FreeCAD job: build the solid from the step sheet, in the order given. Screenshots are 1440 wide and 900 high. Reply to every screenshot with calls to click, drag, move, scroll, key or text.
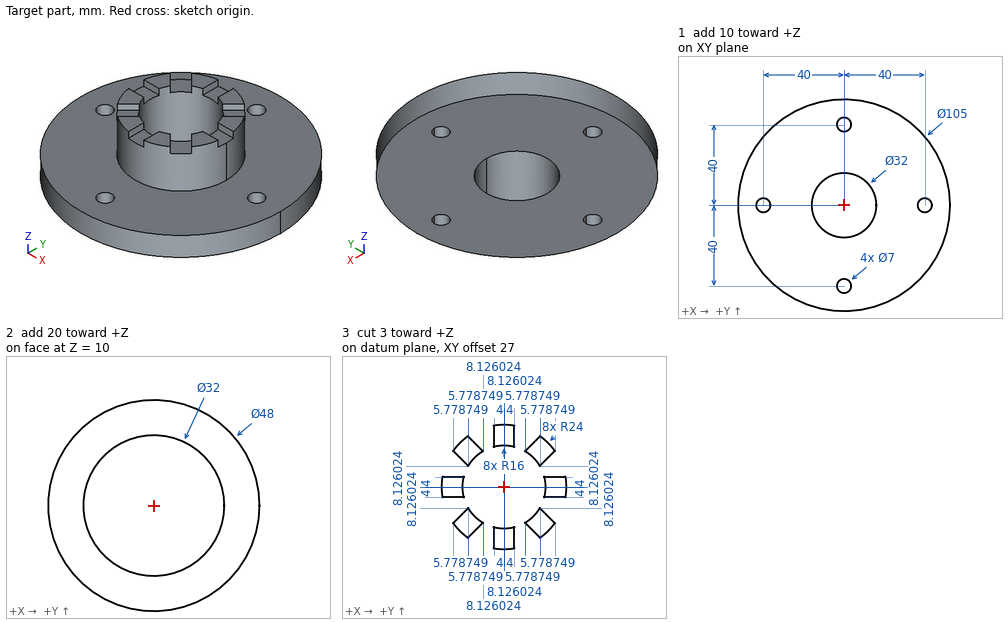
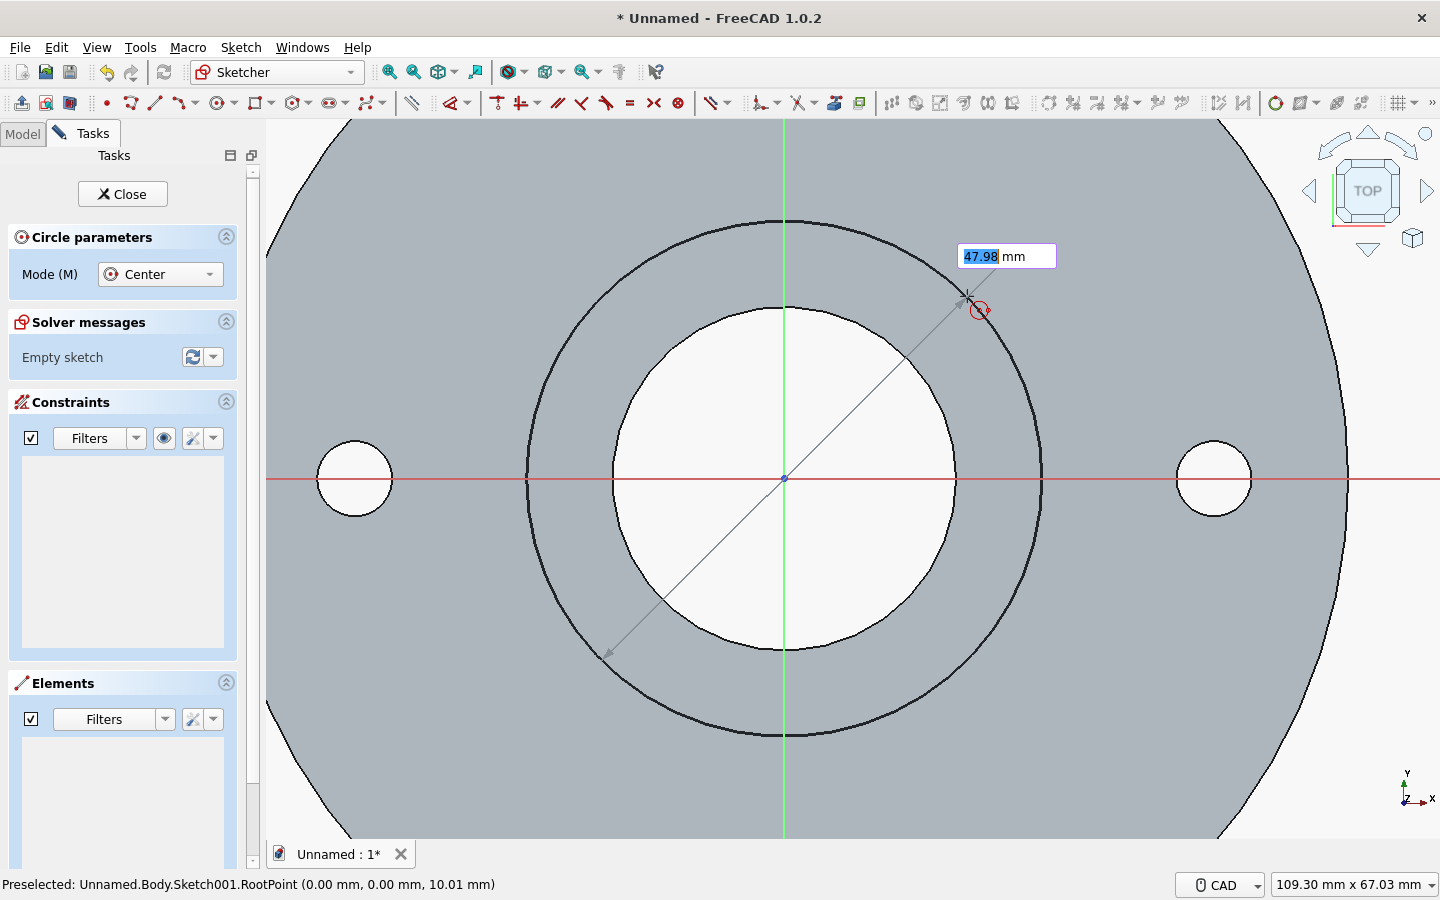
text(48)
key(Return)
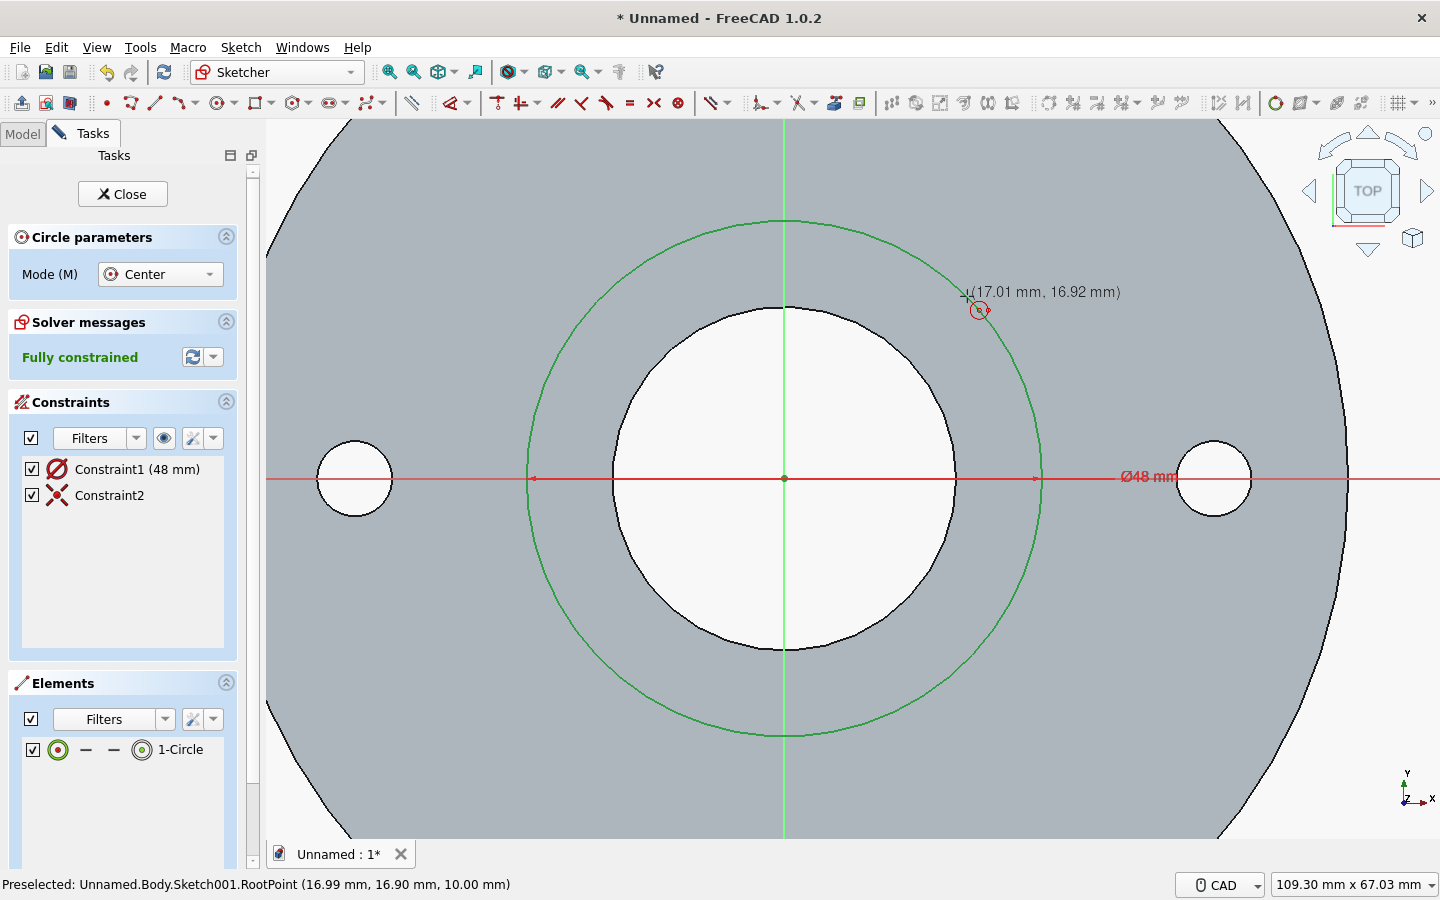
click(784, 479)
move(906, 357)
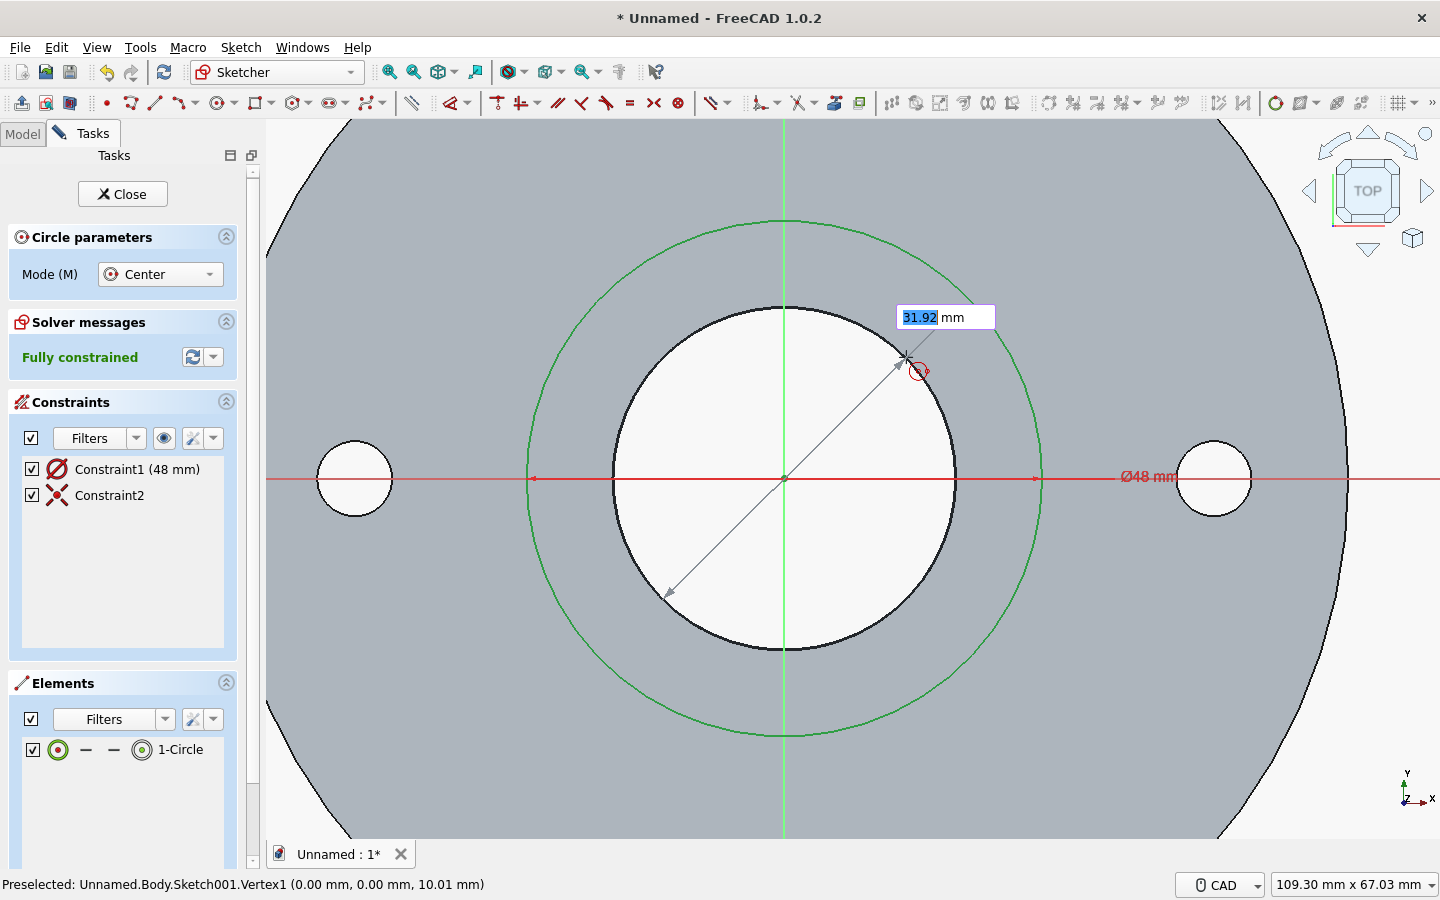
text(32)
key(Return)
key(Escape)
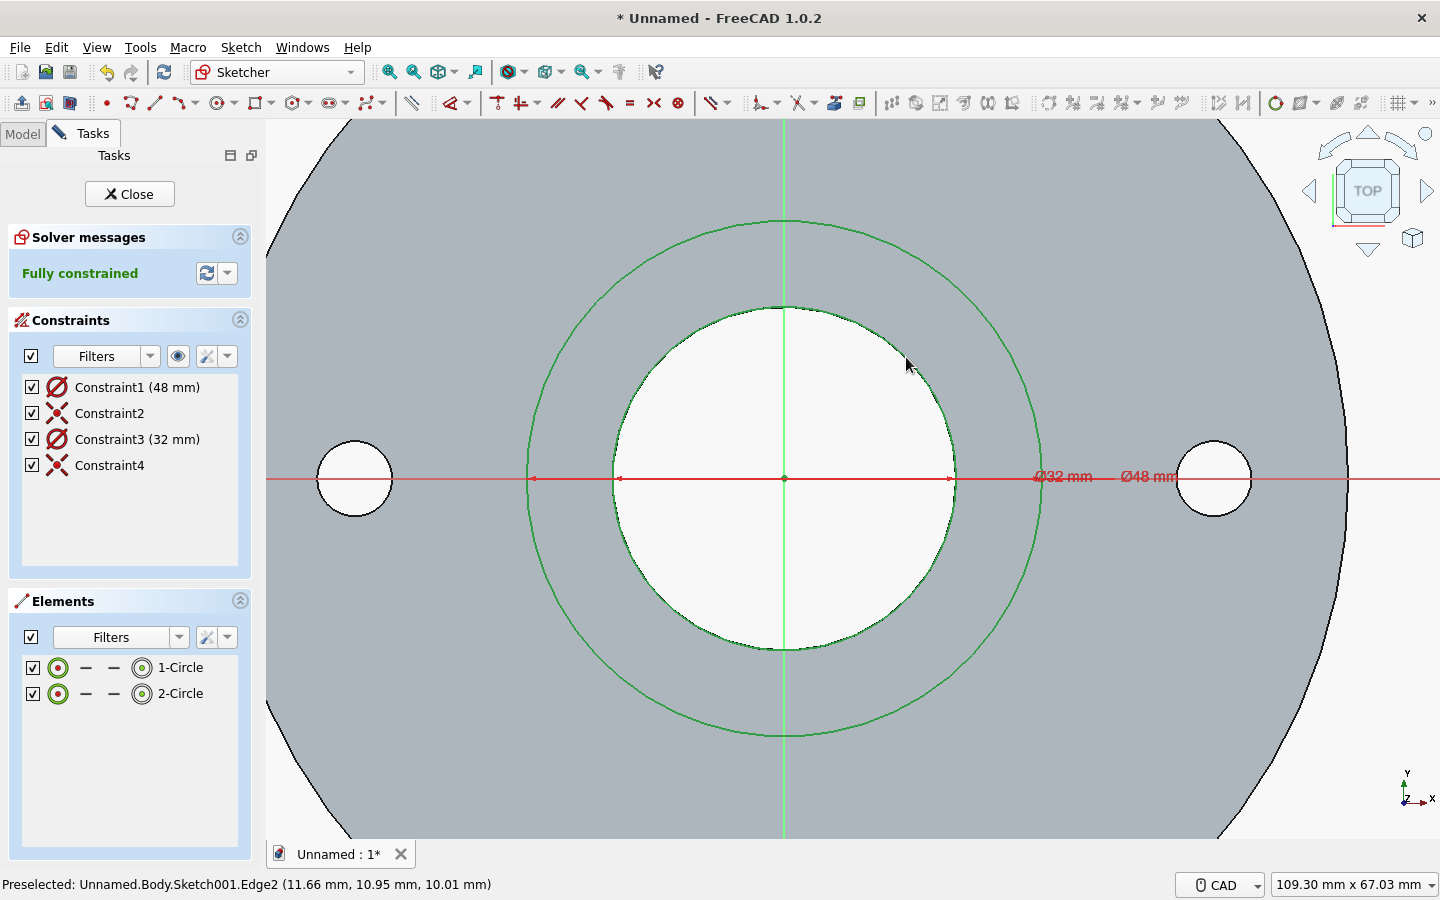
click(130, 194)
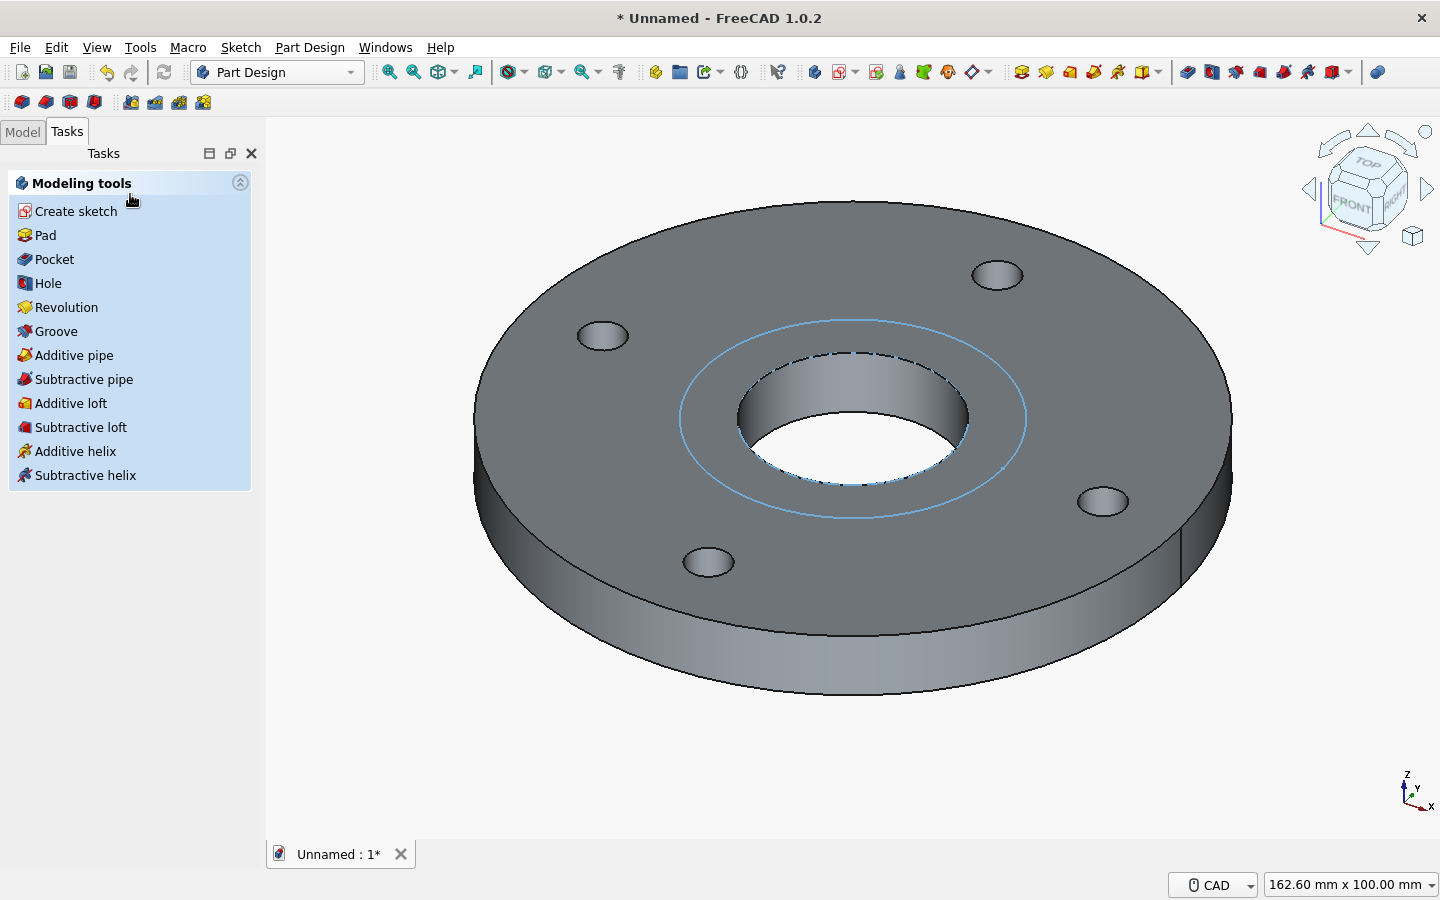
click(1022, 72)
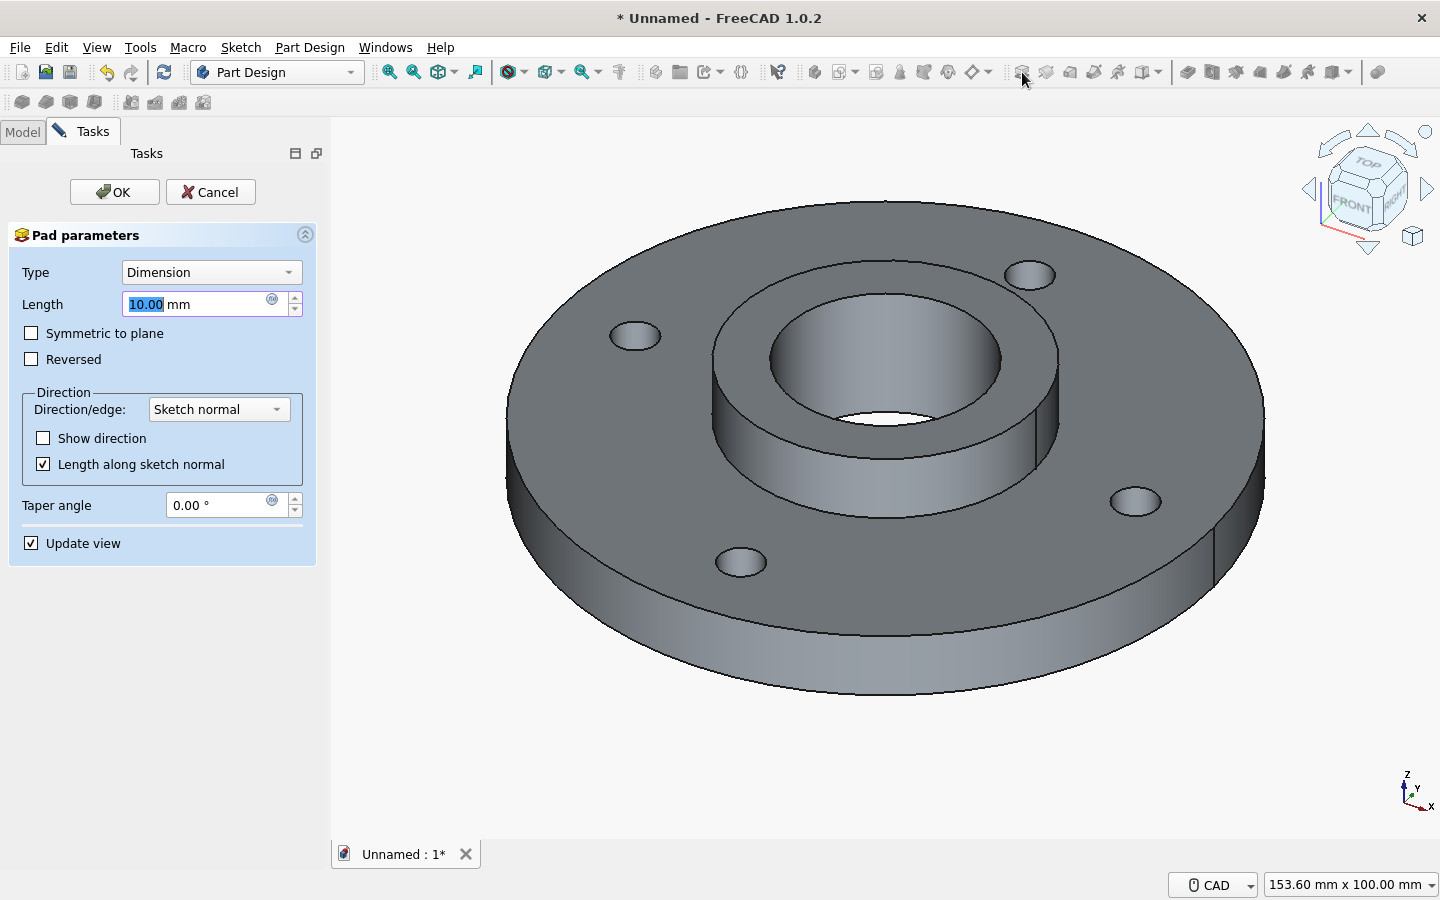
text(20)
key(Tab)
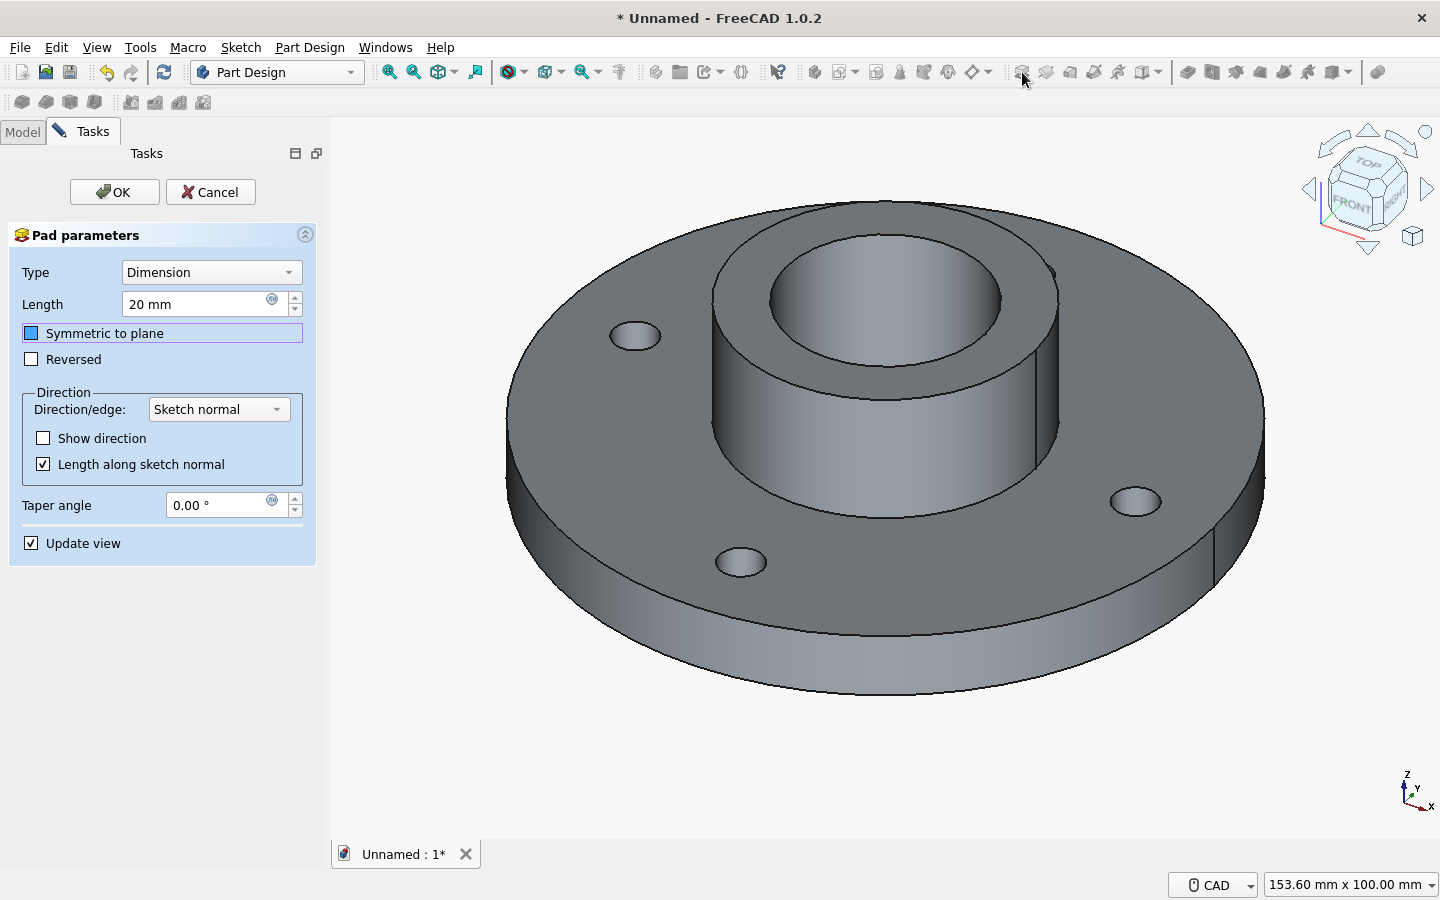
click(115, 192)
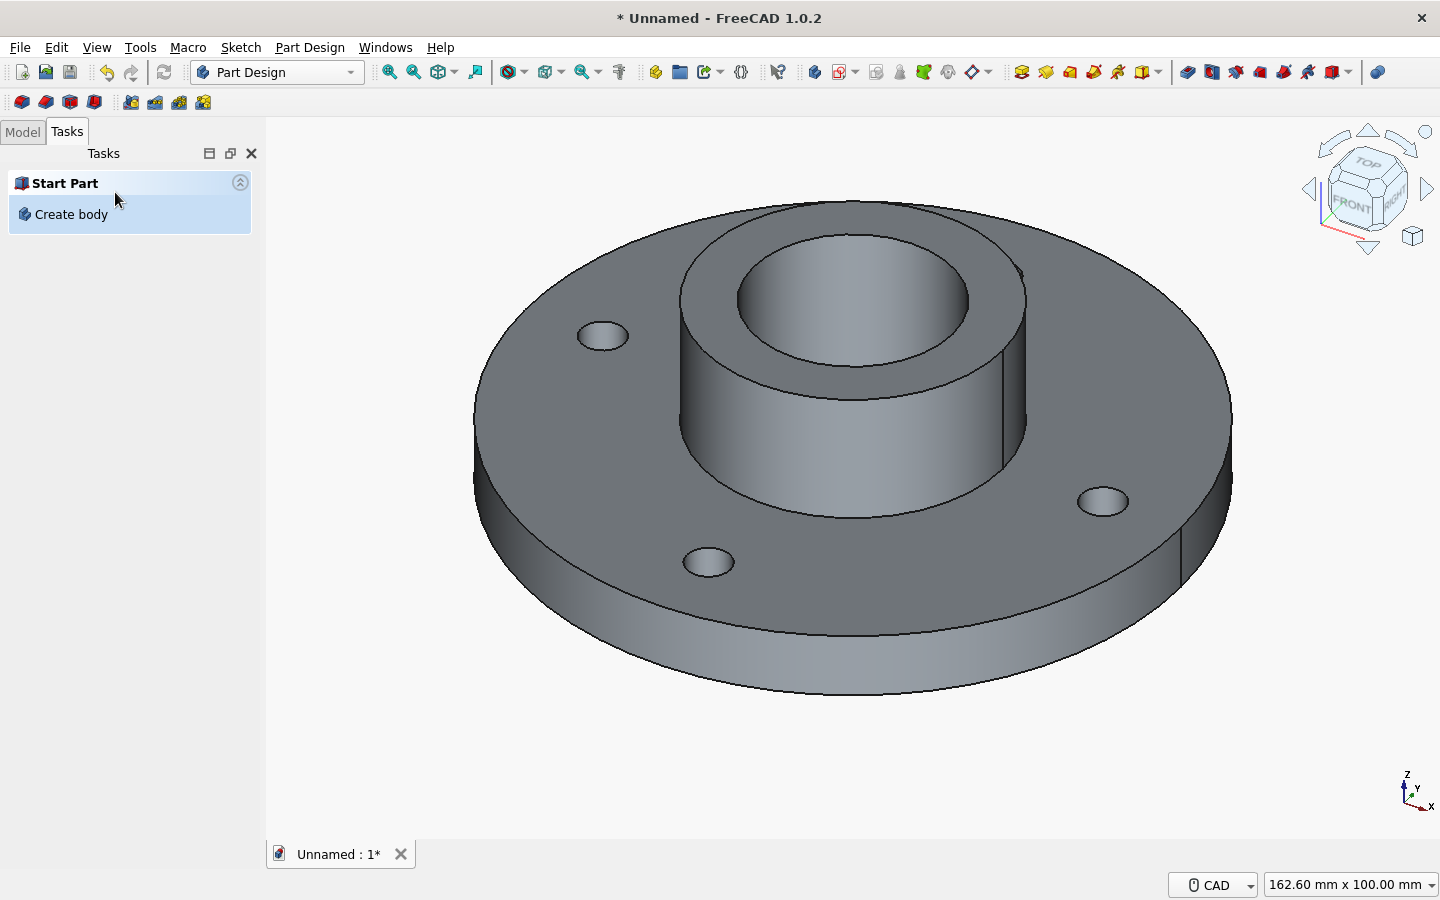
click(390, 72)